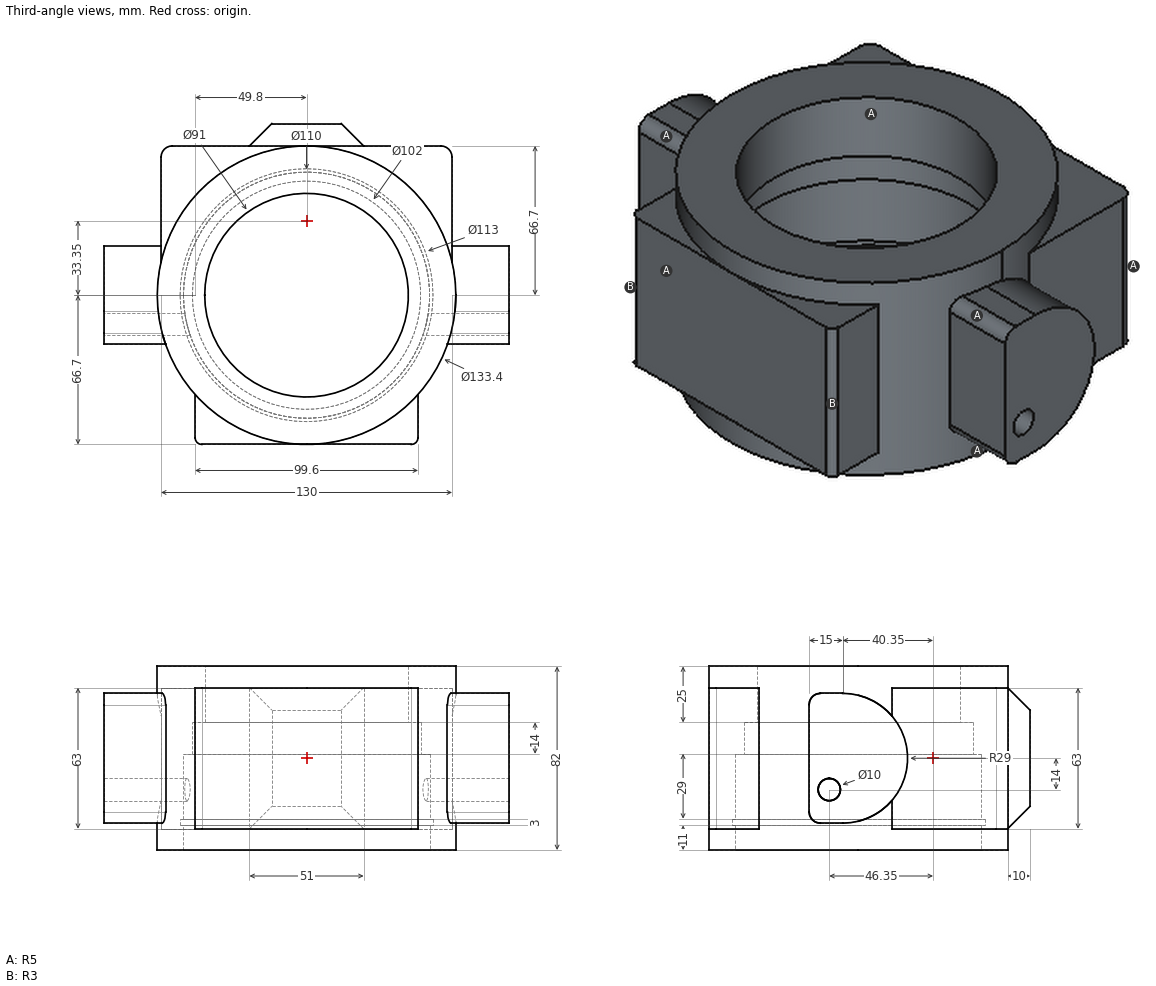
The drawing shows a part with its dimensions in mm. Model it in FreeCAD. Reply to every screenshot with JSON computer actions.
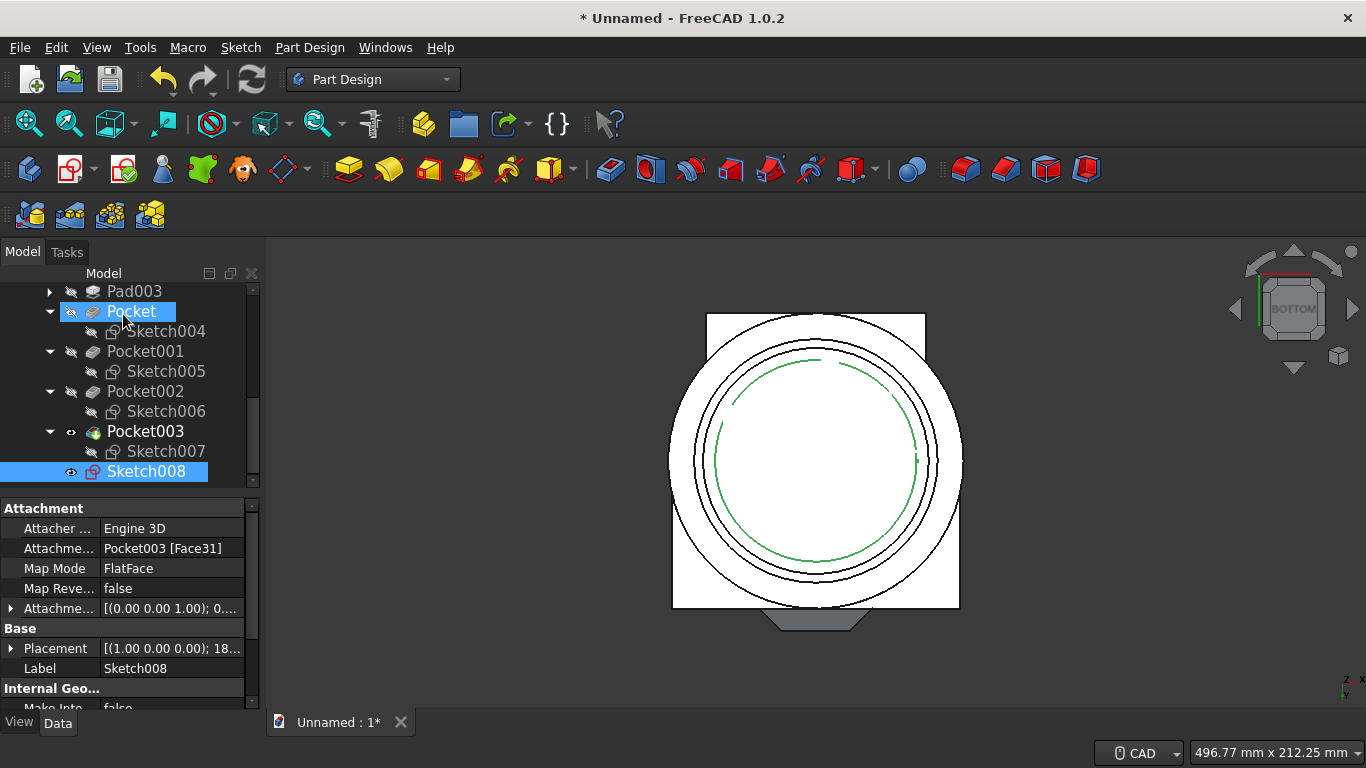
{"action": "left_click", "coordinate": [612, 170]}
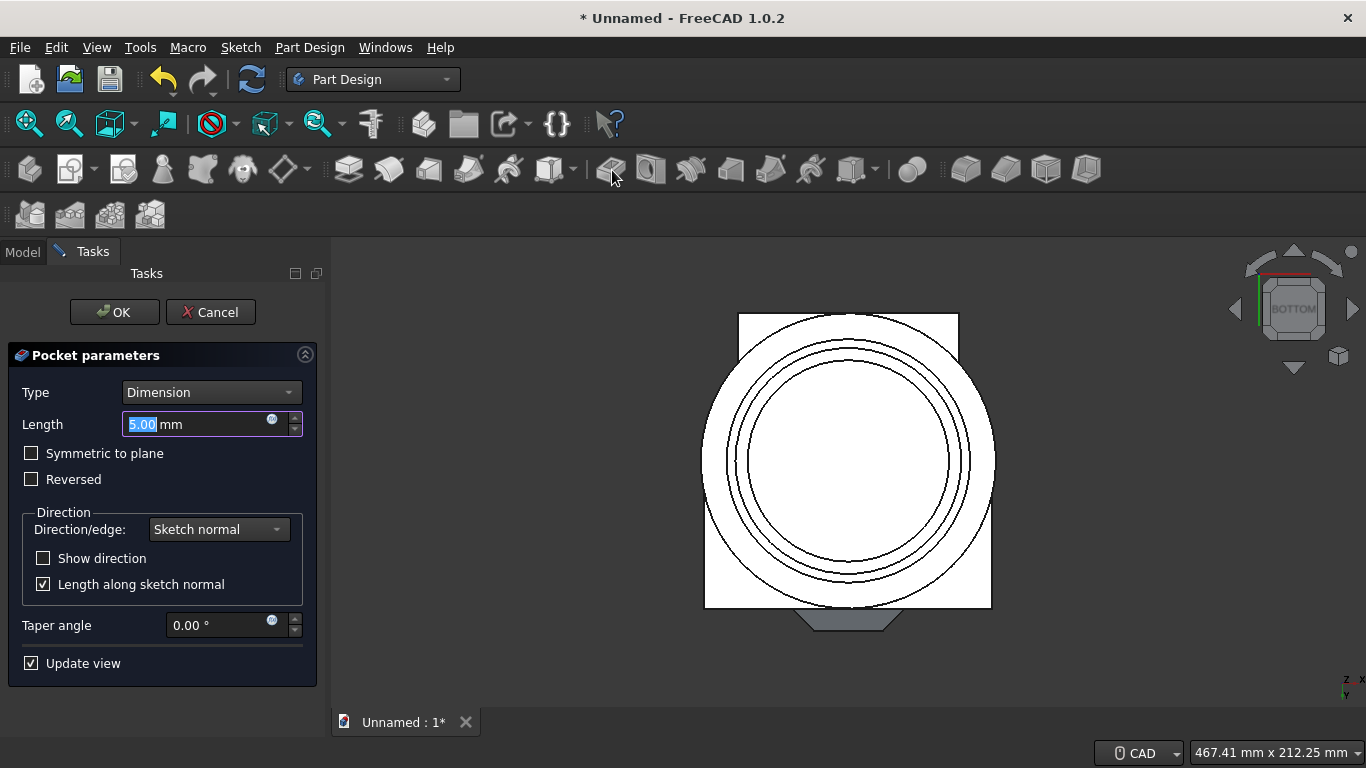
{"action": "type", "text": "25"}
{"action": "key", "text": "Tab"}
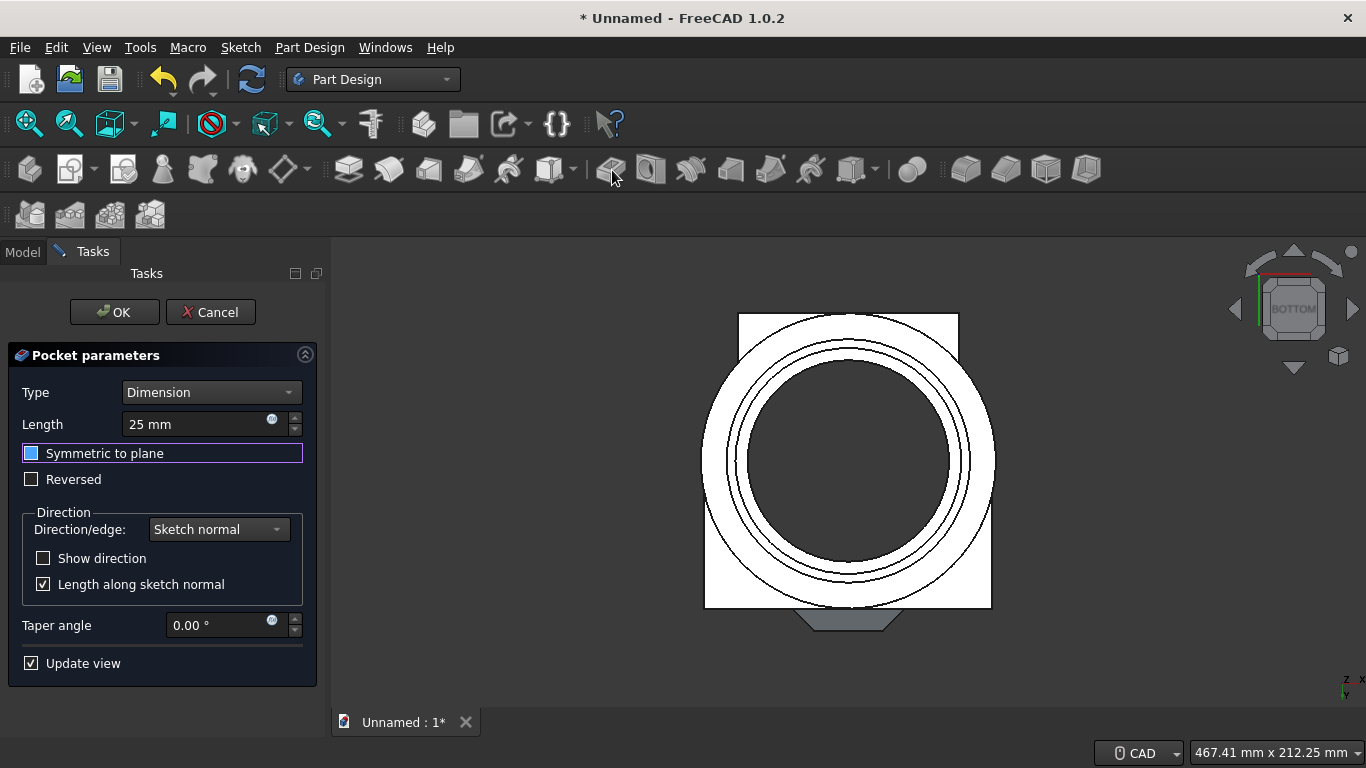
{"action": "left_click", "coordinate": [115, 312]}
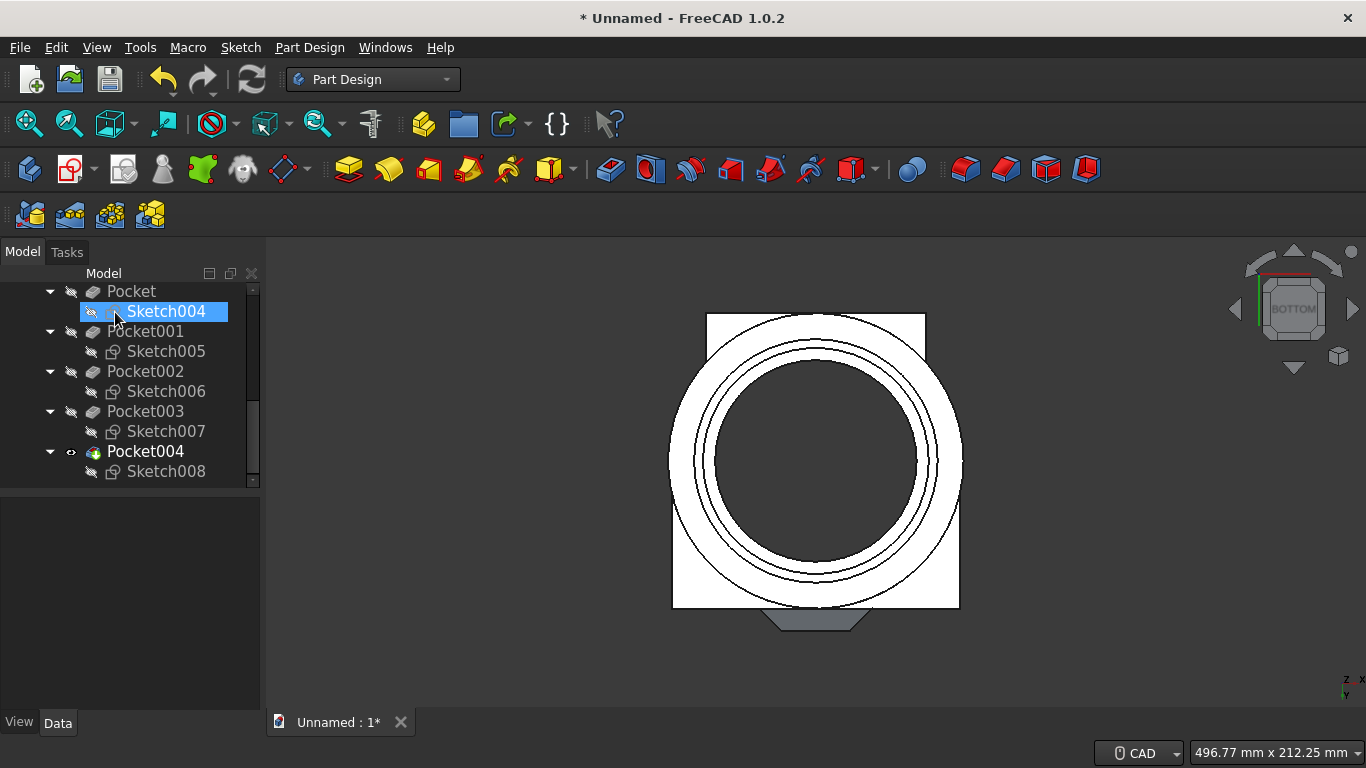
{"action": "scroll", "coordinate": [140, 387], "scroll_direction": "down", "scroll_amount": 3}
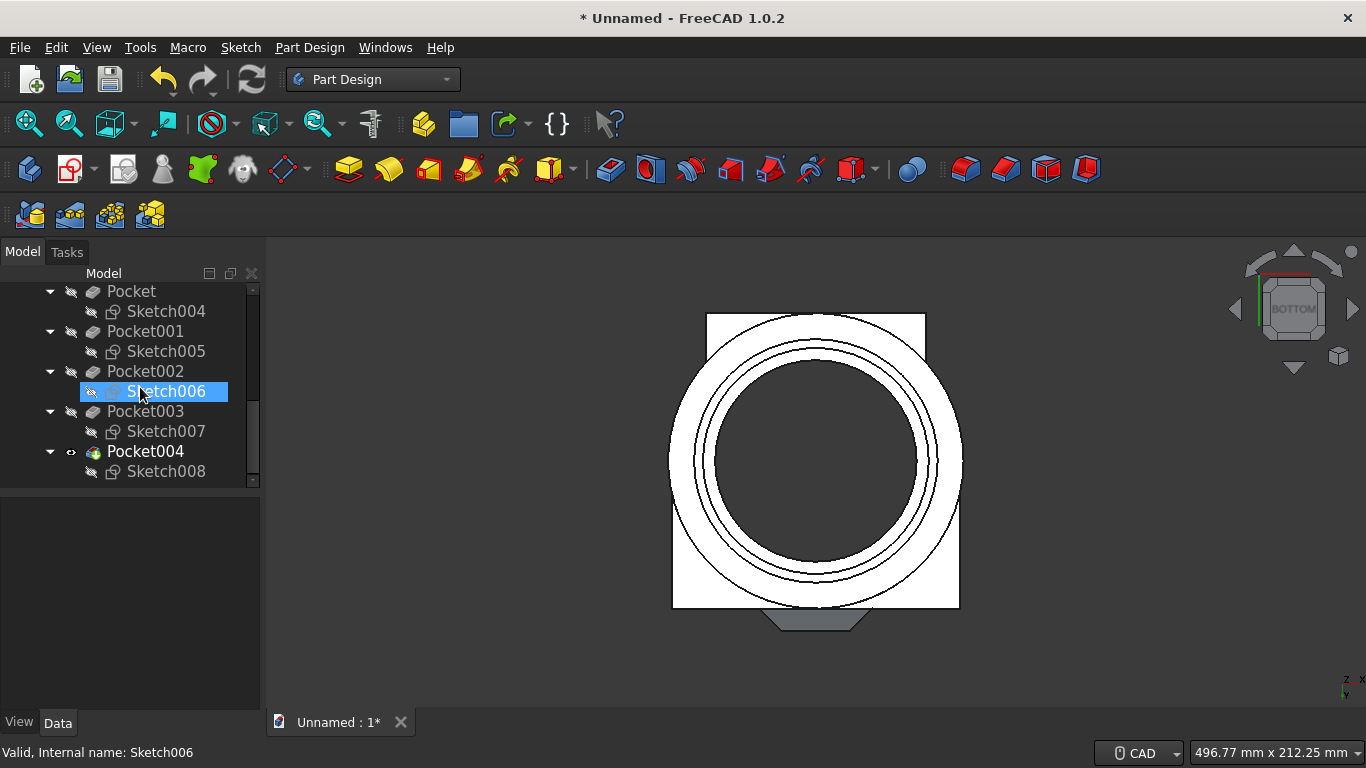
{"action": "scroll", "coordinate": [140, 387], "scroll_direction": "up", "scroll_amount": 15}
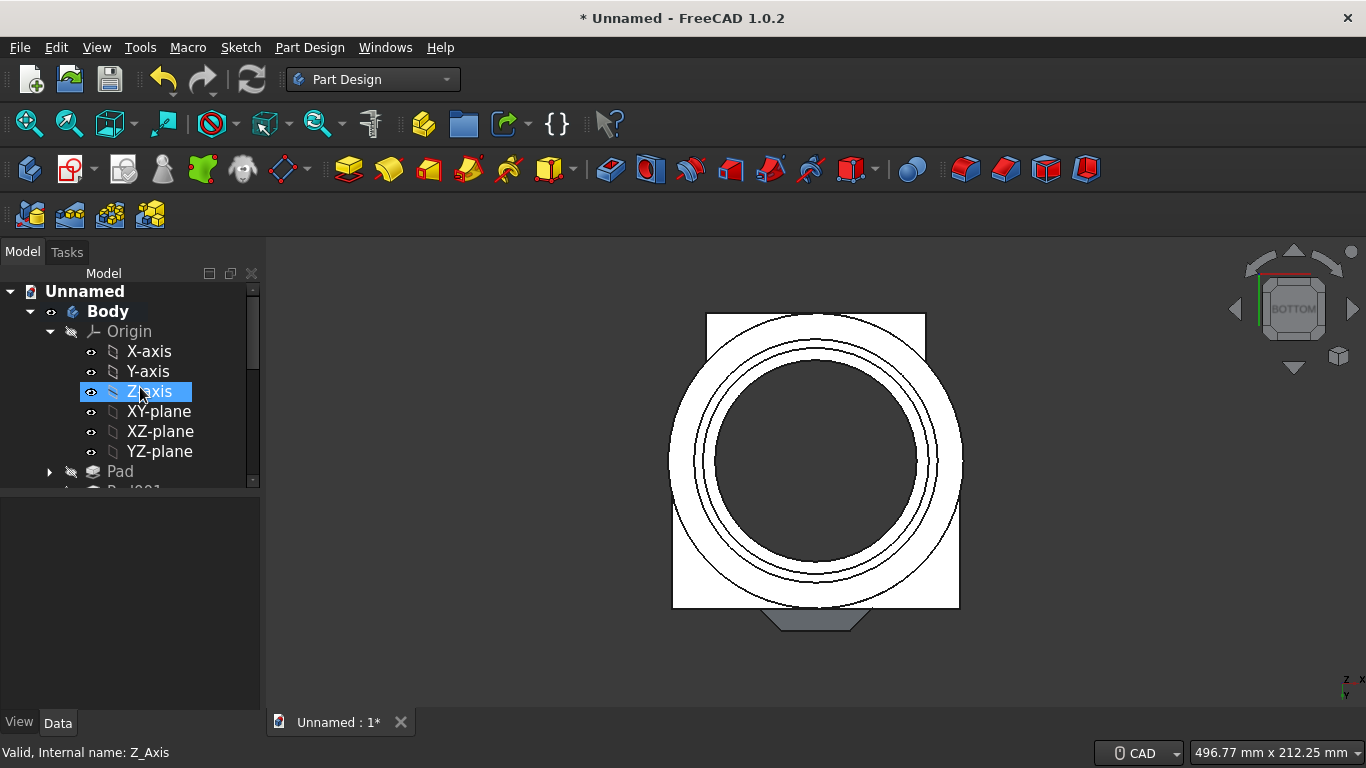
{"action": "left_click", "coordinate": [136, 452]}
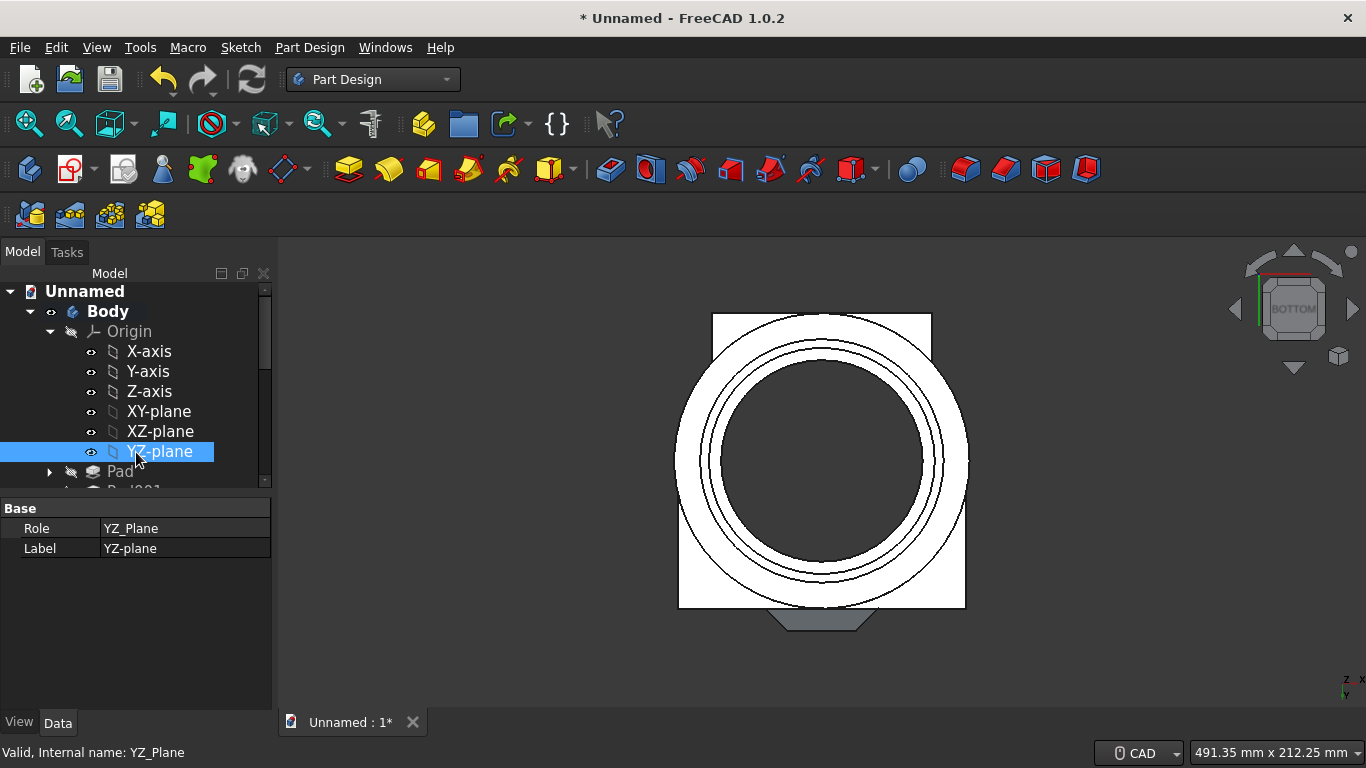
{"action": "left_click", "coordinate": [284, 170]}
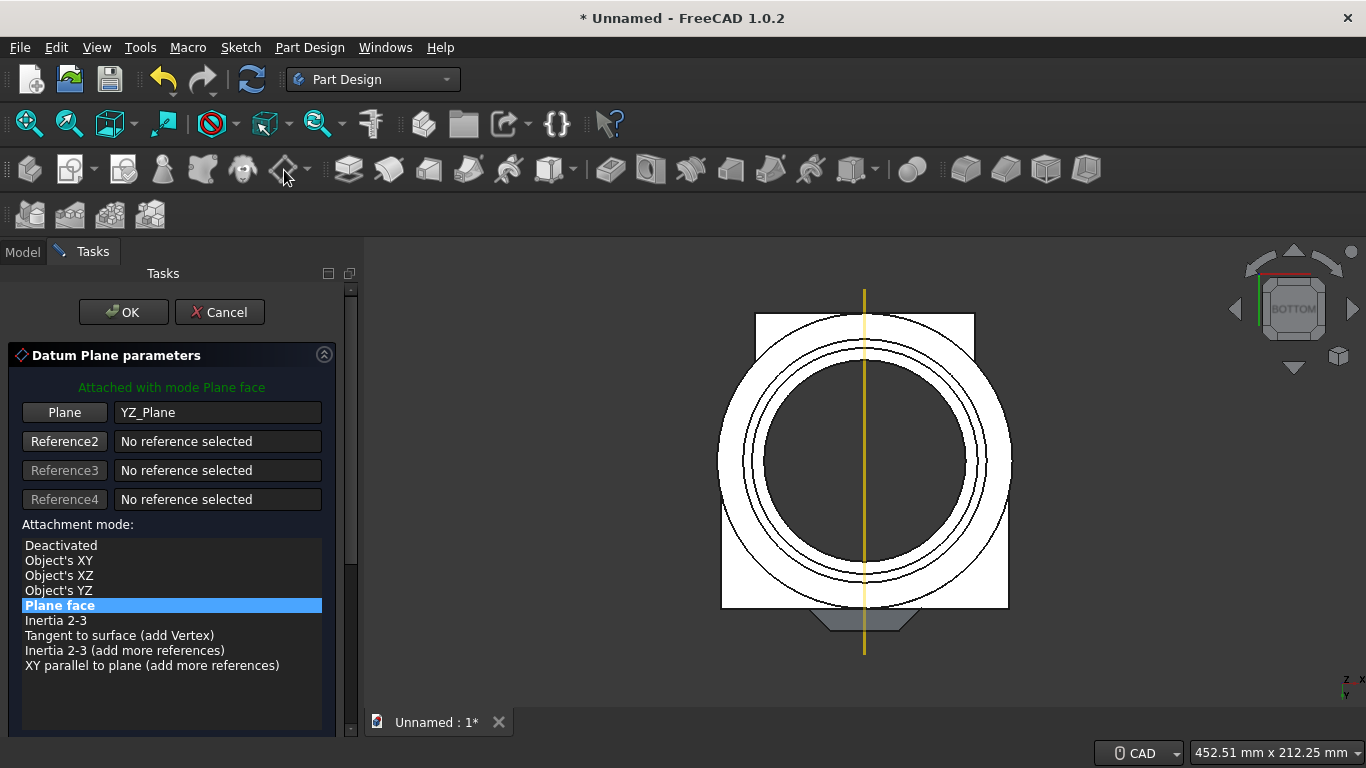
{"action": "scroll", "coordinate": [351, 510], "scroll_direction": "down", "scroll_amount": 3}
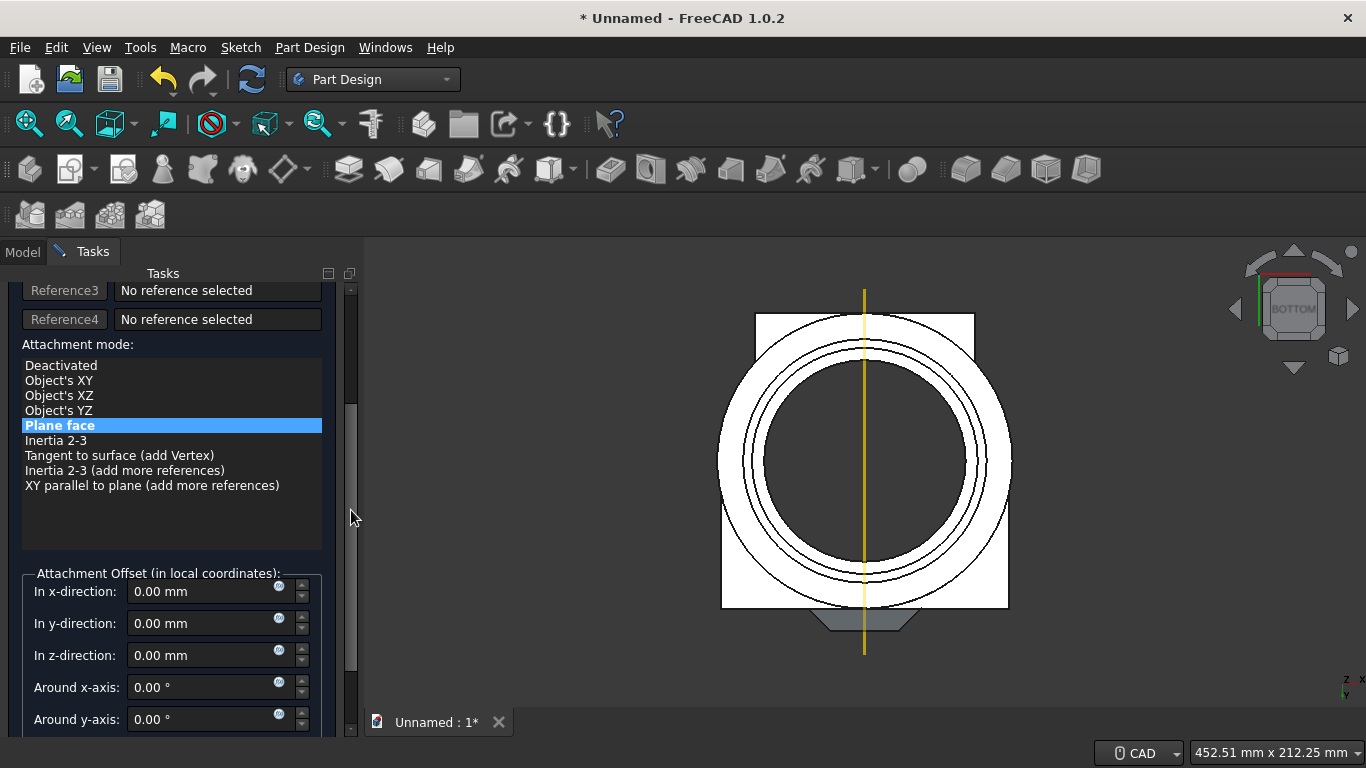
{"action": "triple_click", "coordinate": [210, 655]}